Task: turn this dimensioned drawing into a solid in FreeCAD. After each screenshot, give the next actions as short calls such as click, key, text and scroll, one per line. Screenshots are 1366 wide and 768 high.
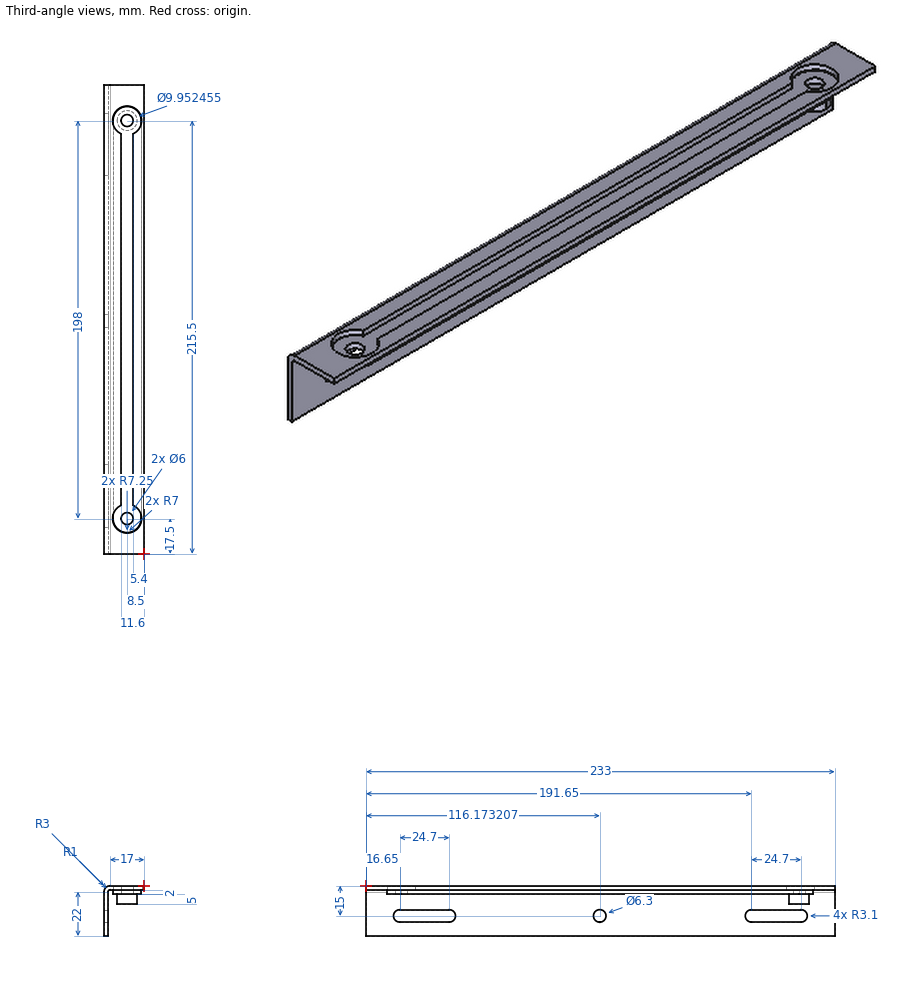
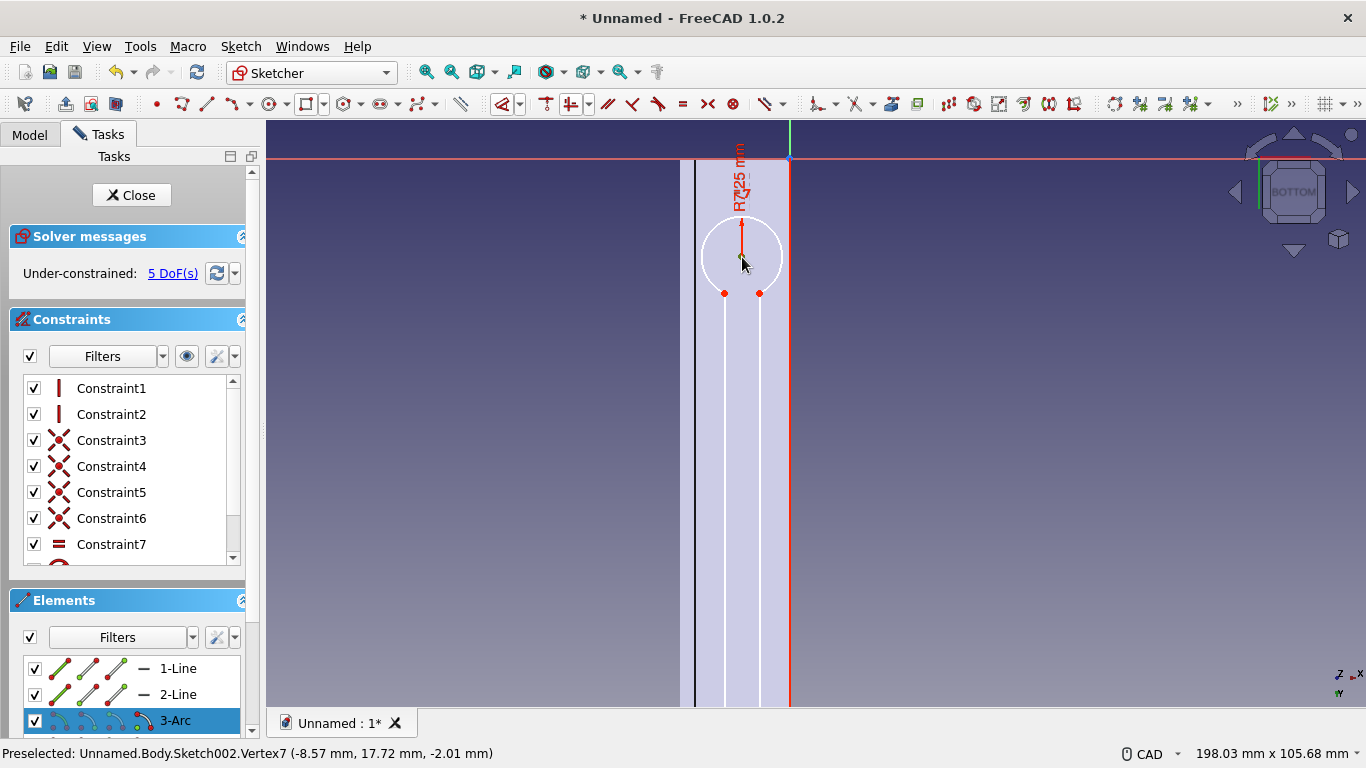
key(l)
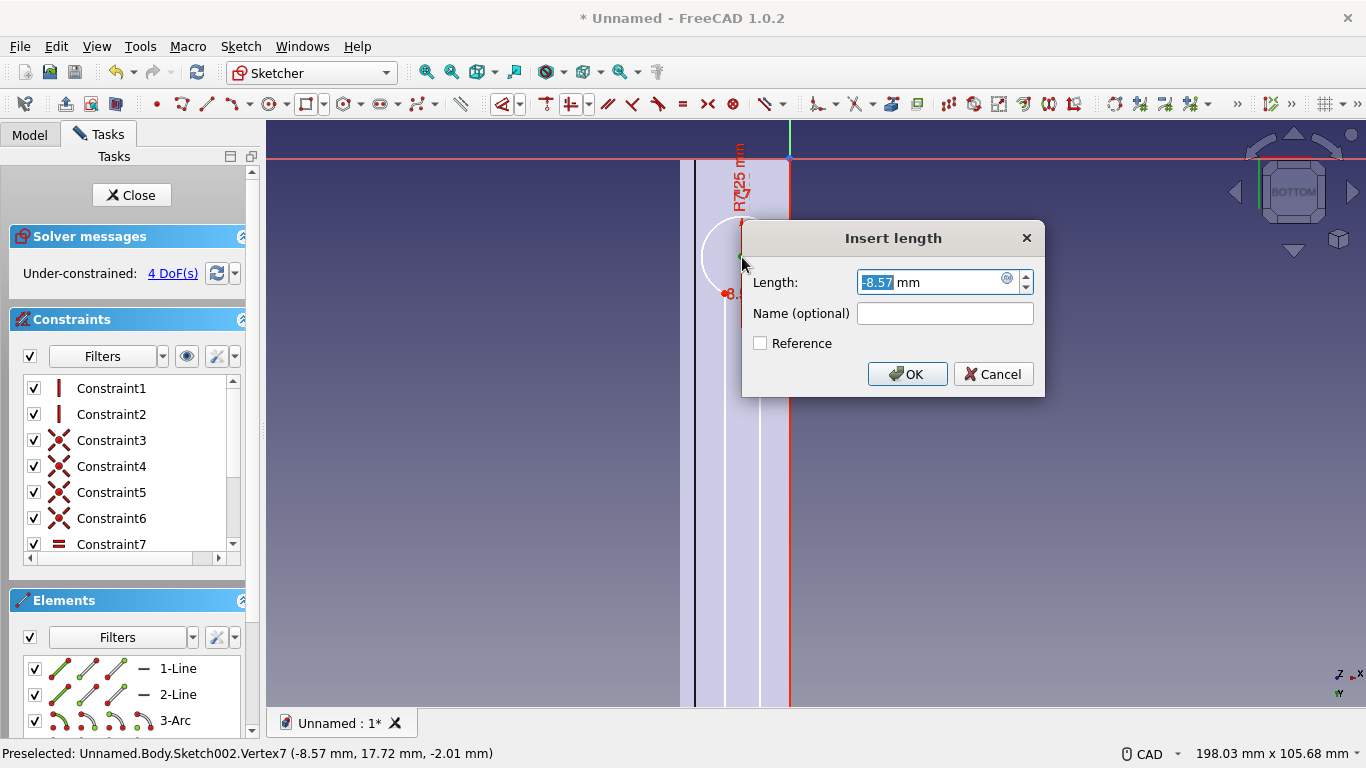
text(-8.5)
key(Return)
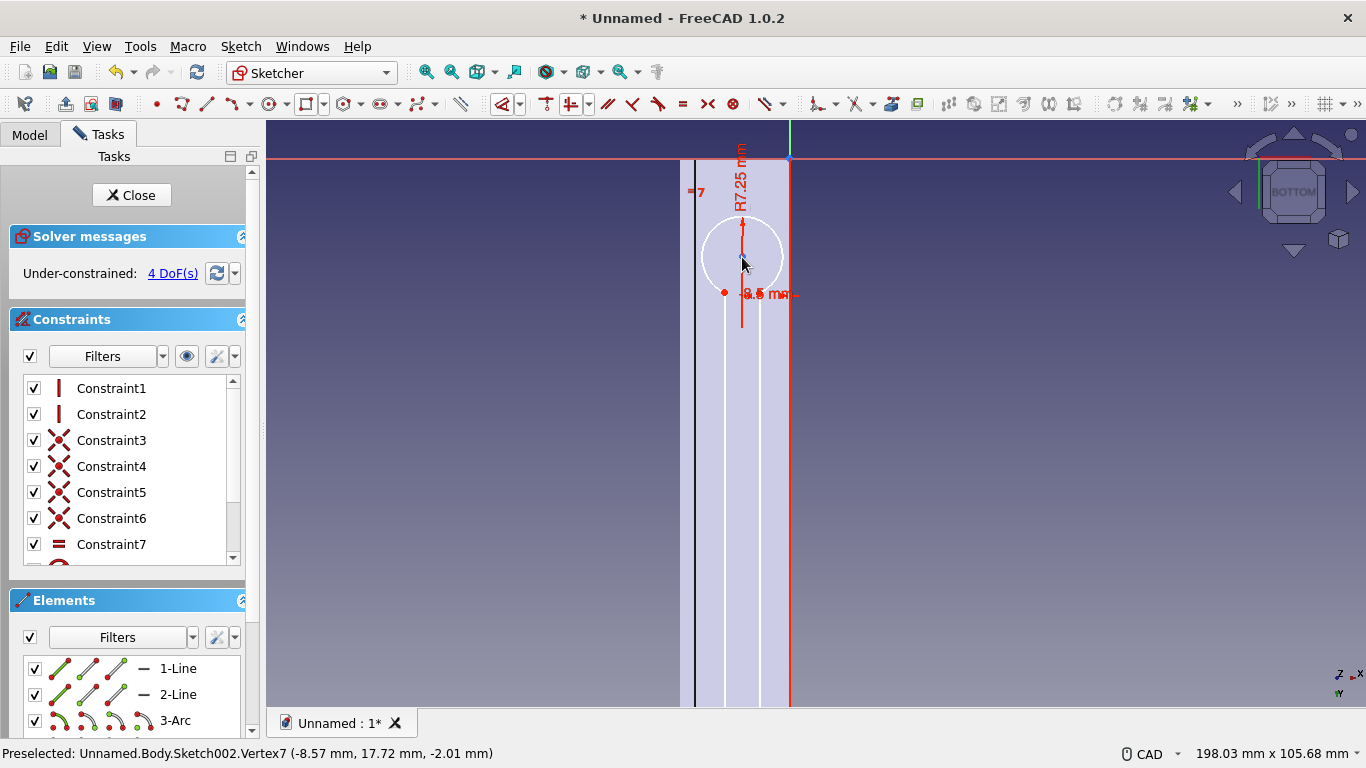
scroll(743, 257, down, 6)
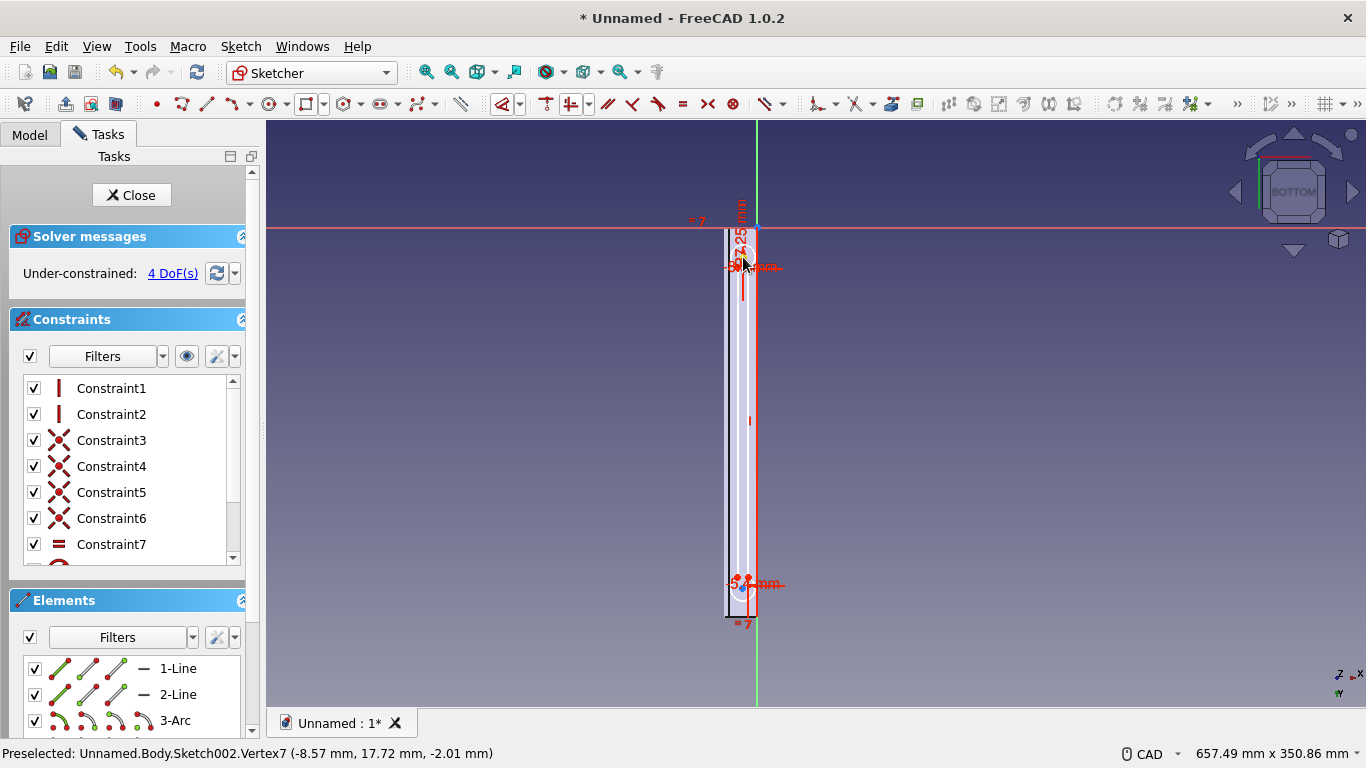
scroll(743, 589, up, 6)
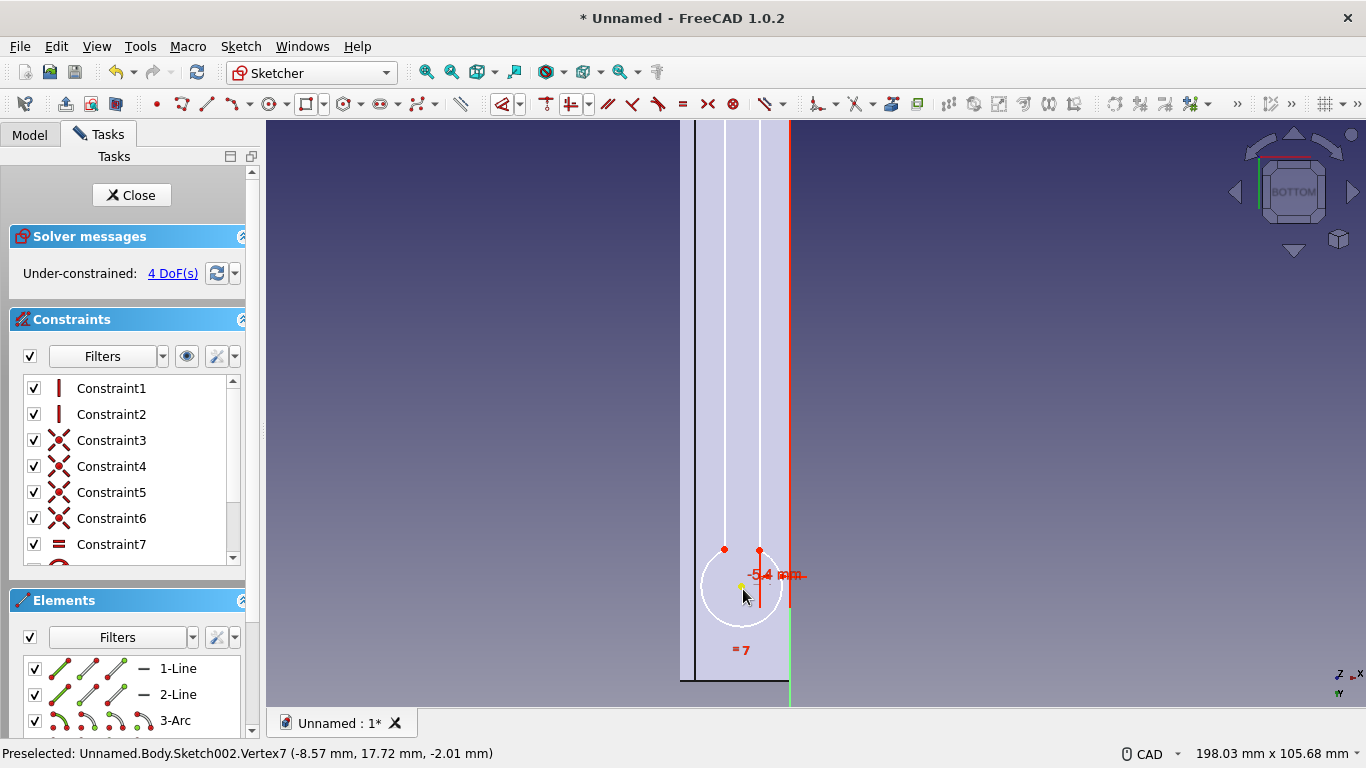
click(742, 586)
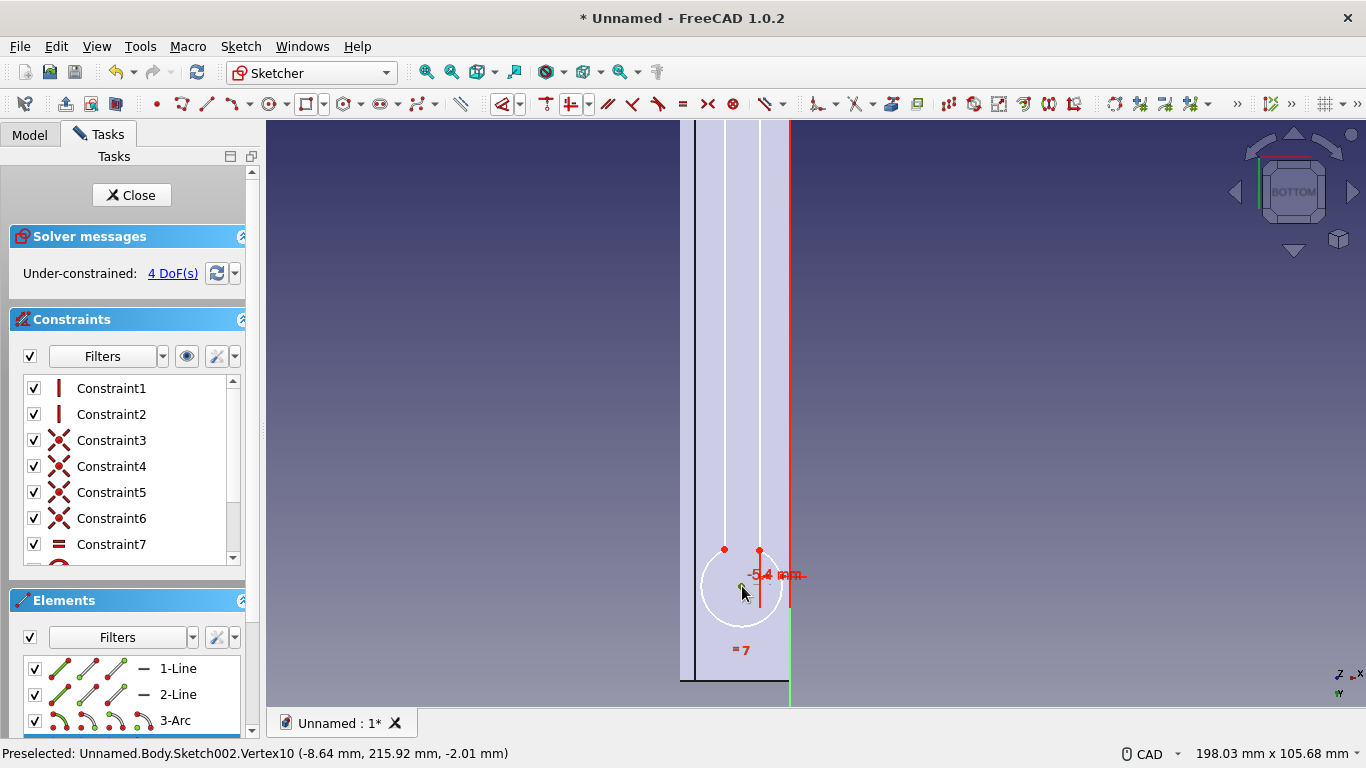
key(l)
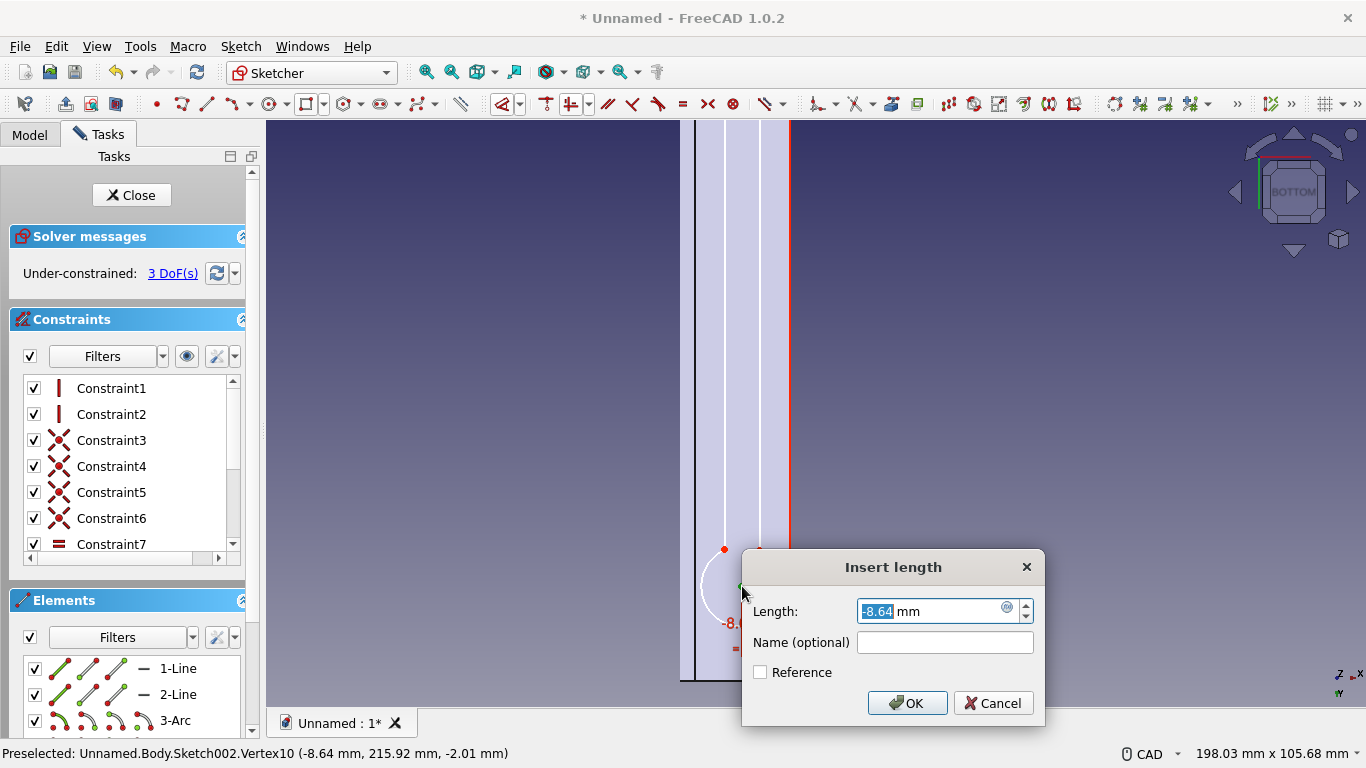
text(-8.5)
key(Return)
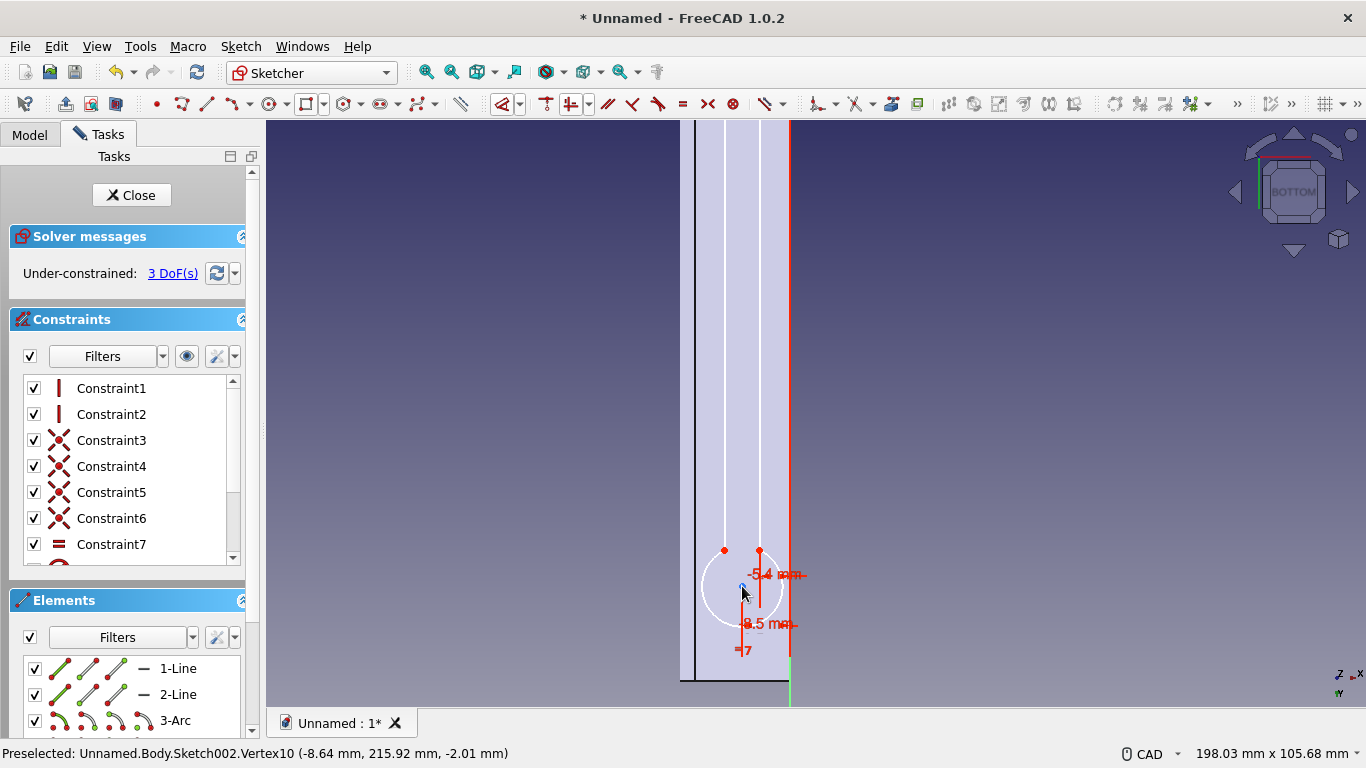
scroll(743, 589, down, 6)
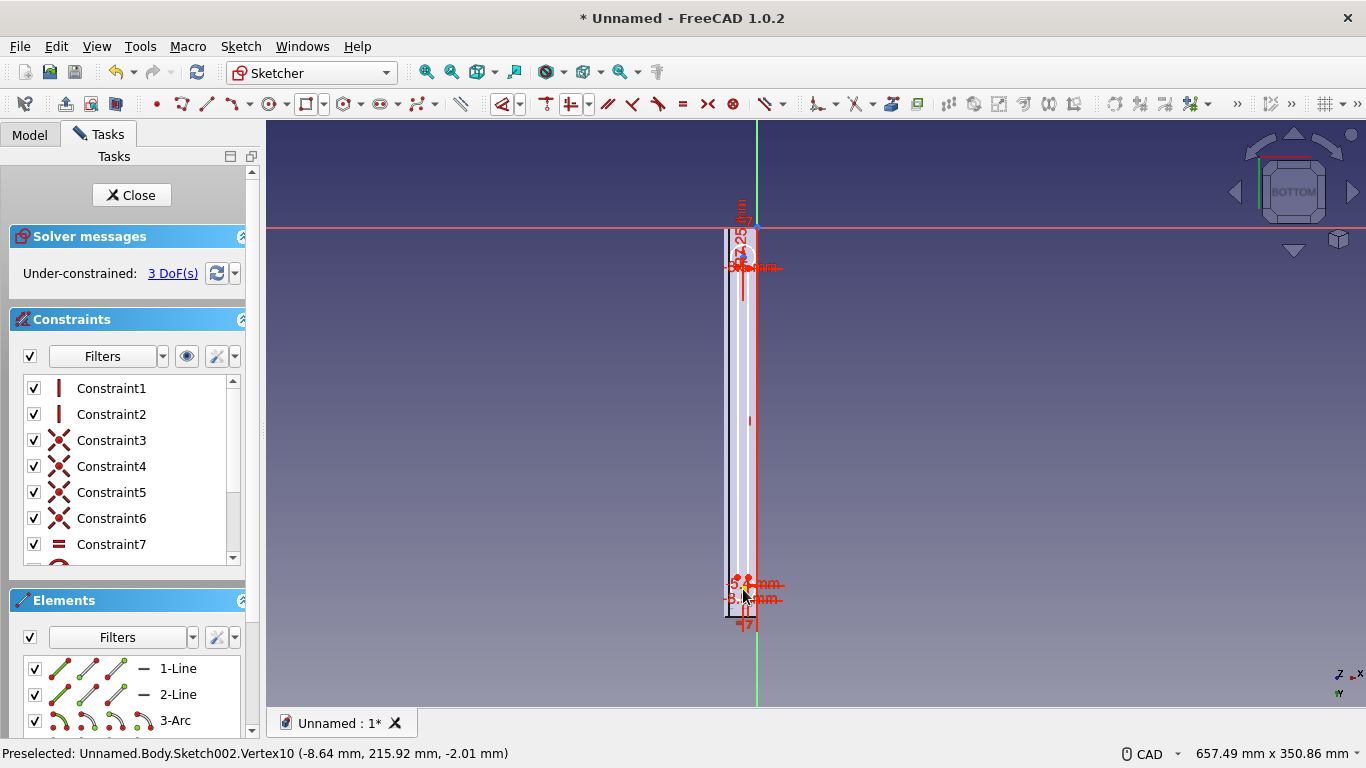
scroll(738, 268, up, 4)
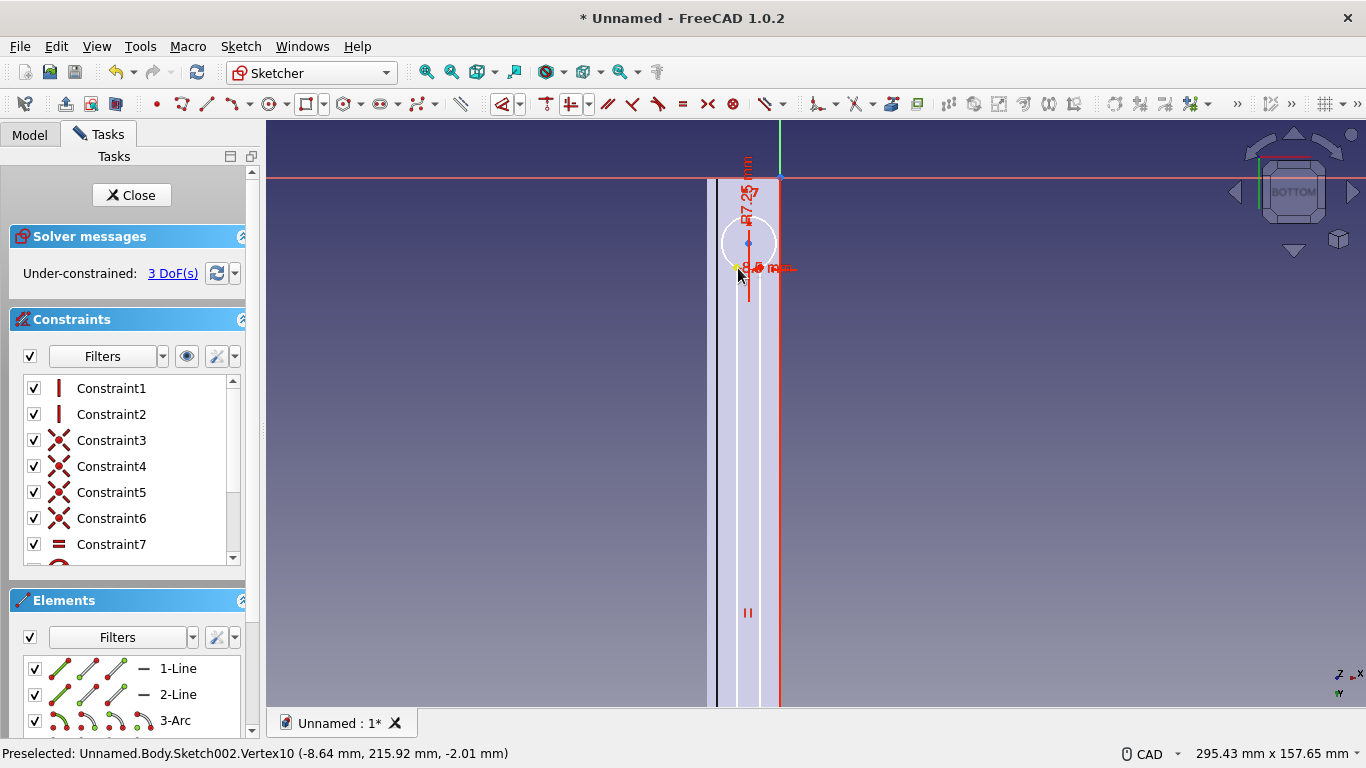
click(737, 268)